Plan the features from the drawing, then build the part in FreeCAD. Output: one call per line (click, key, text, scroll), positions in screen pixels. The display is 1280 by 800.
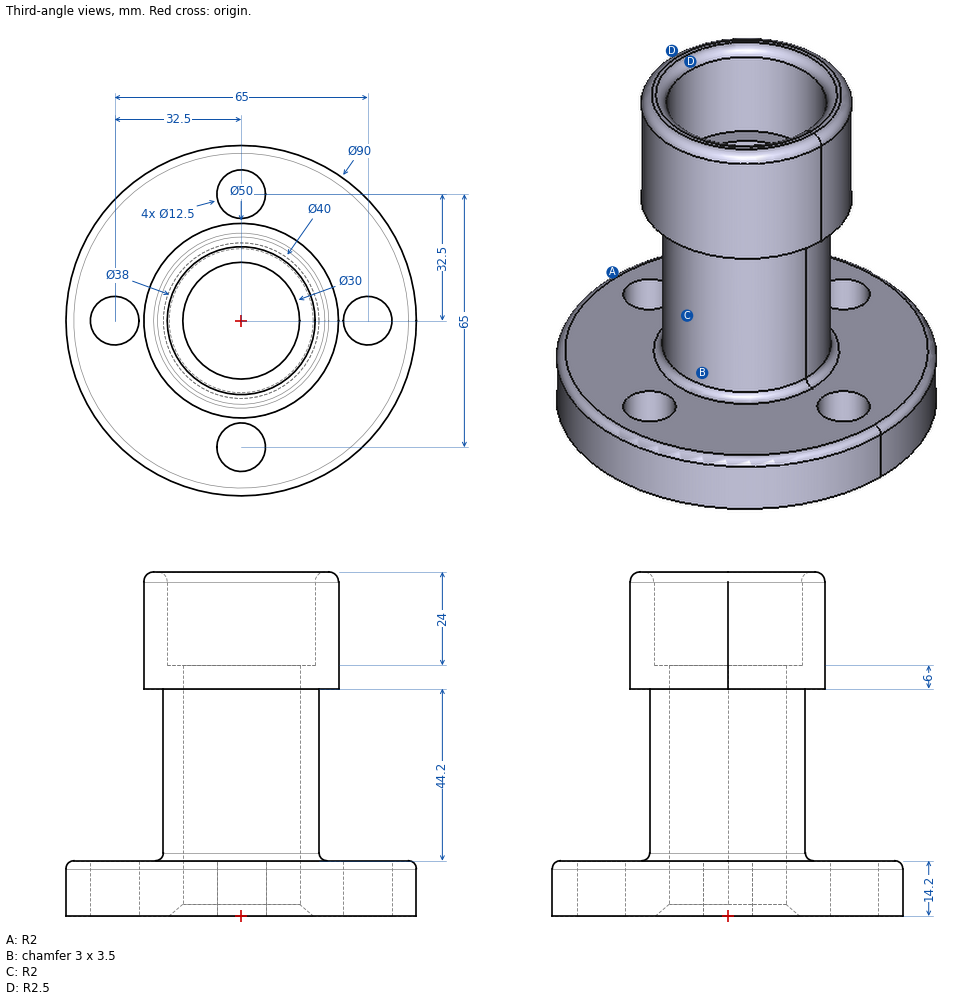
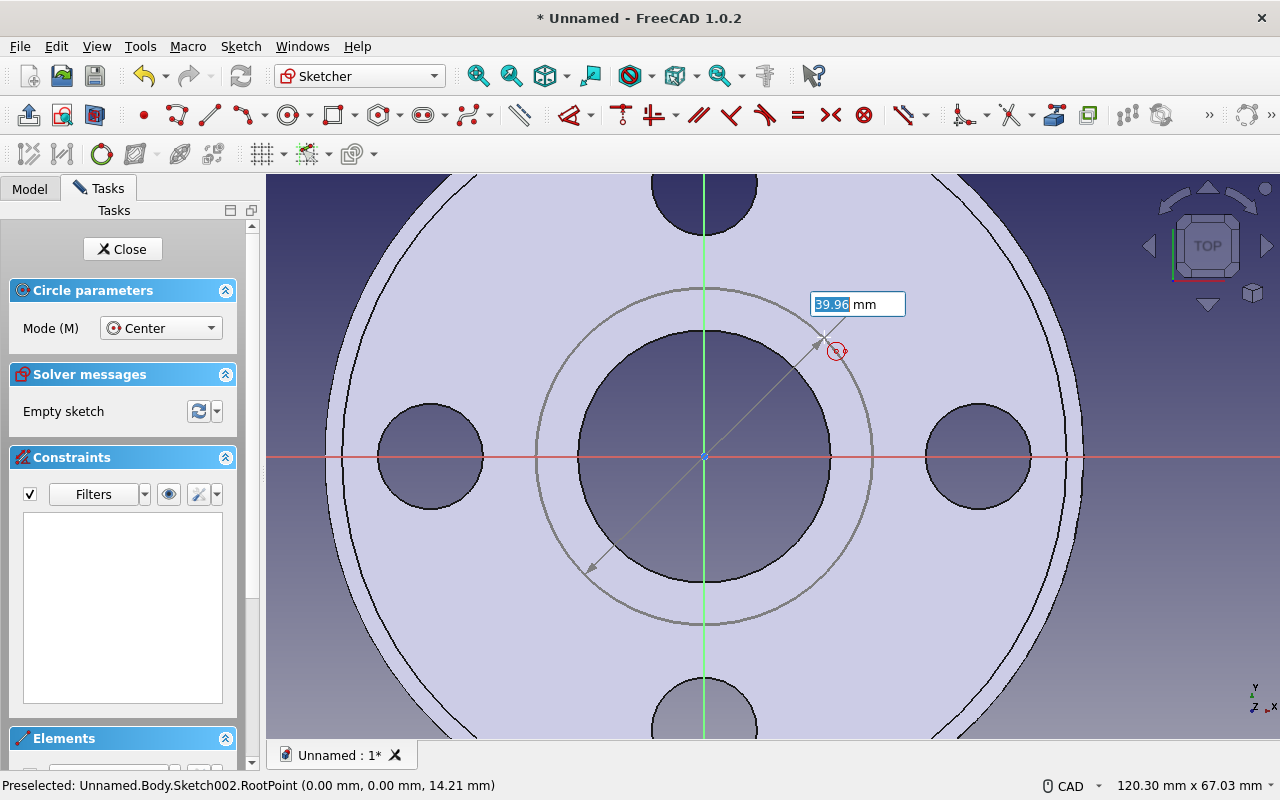
text(40)
key(Return)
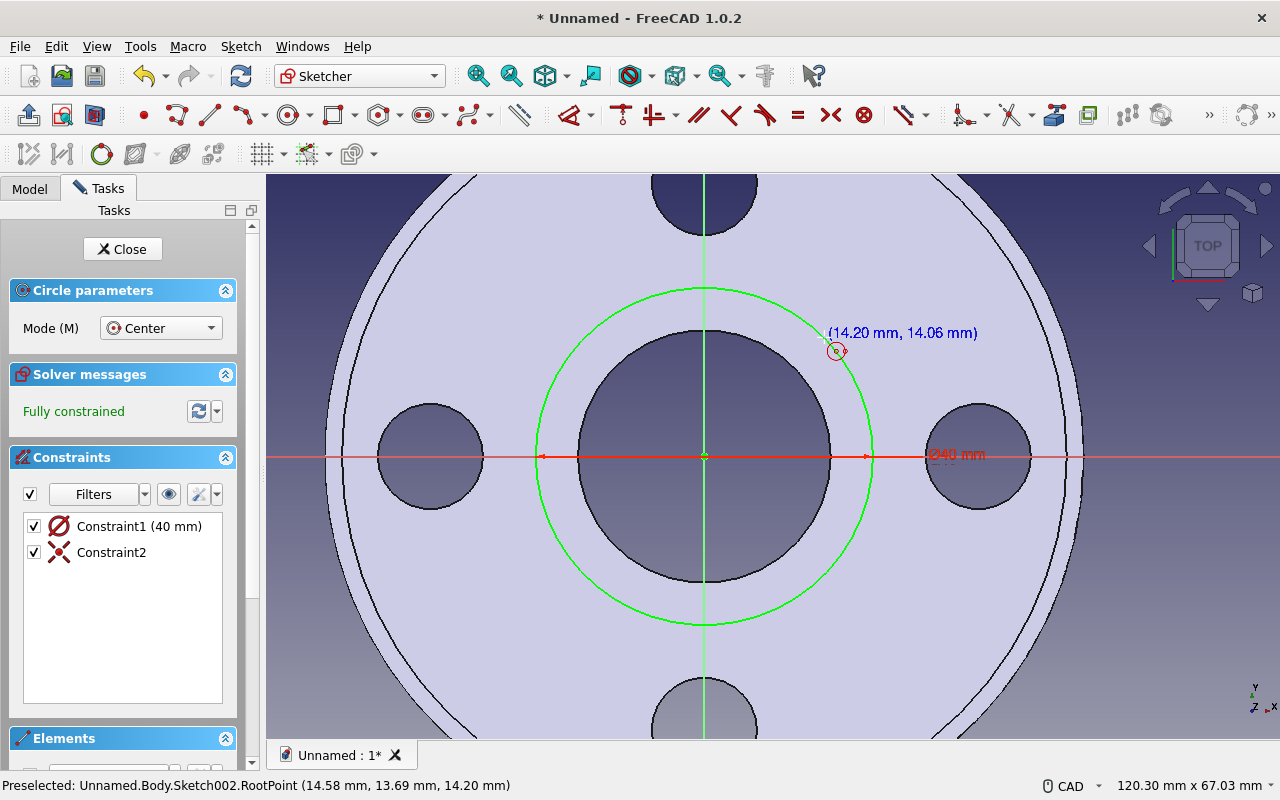
click(704, 456)
move(794, 367)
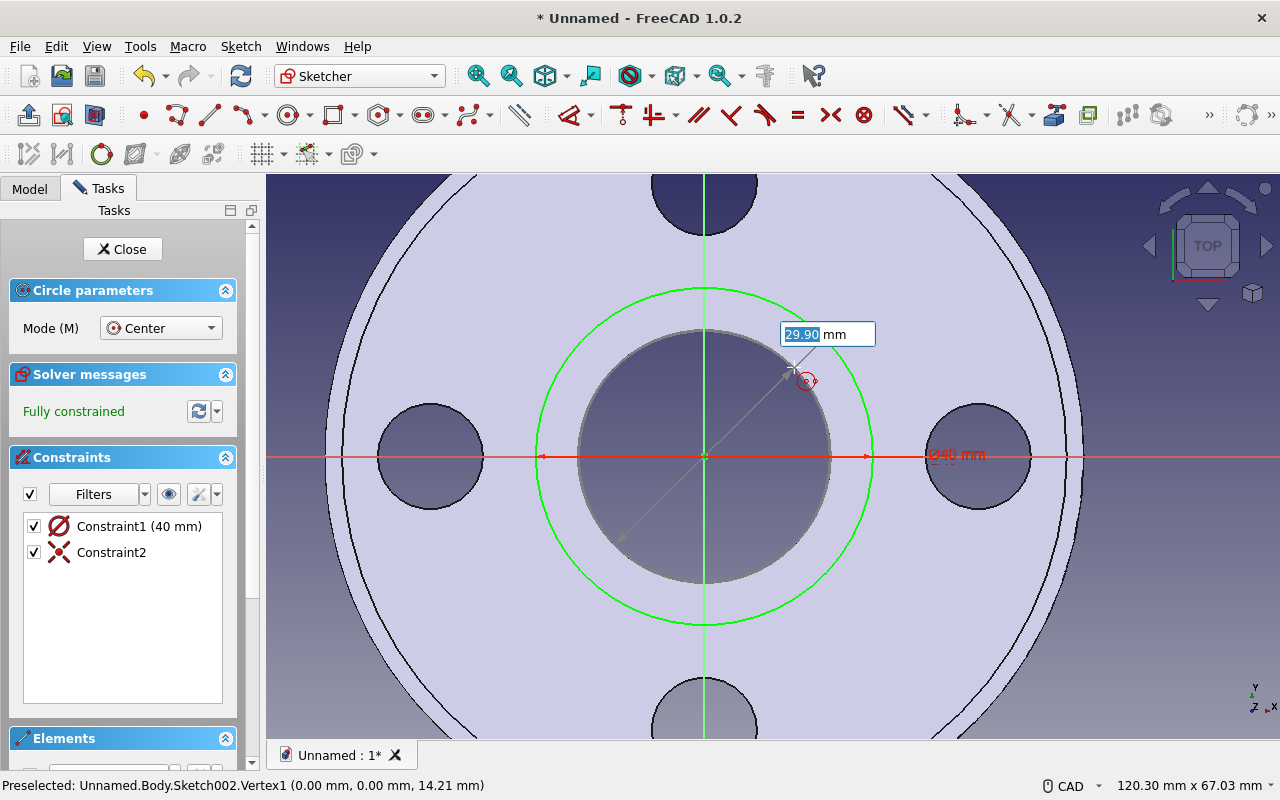
text(30)
key(Return)
key(Escape)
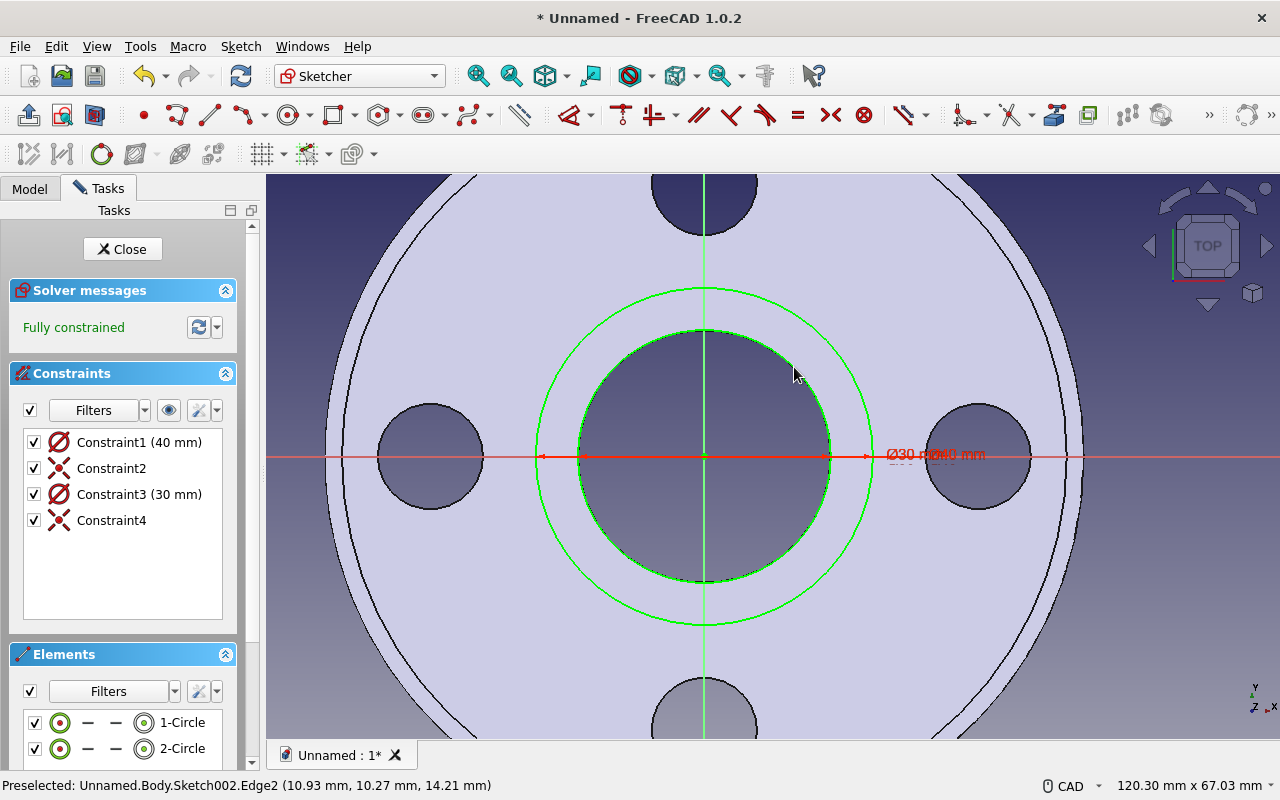
click(123, 249)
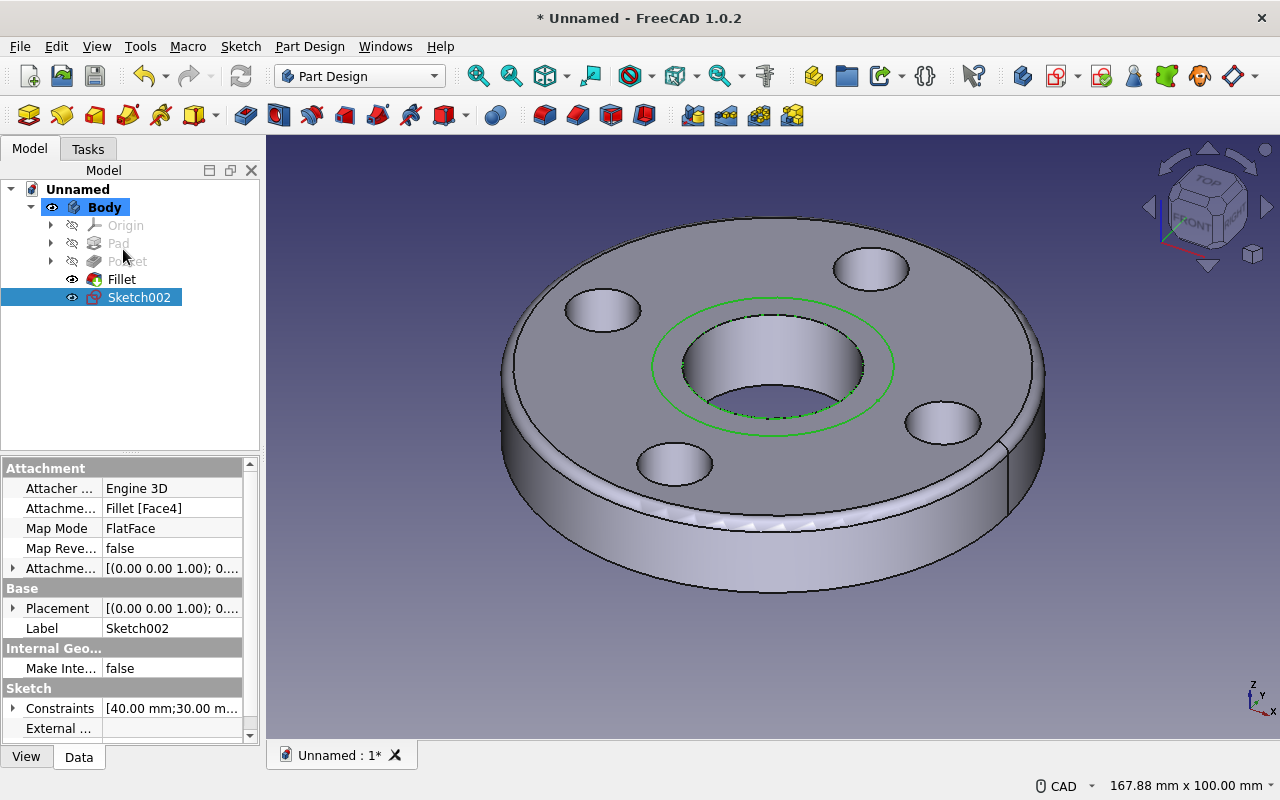
click(29, 116)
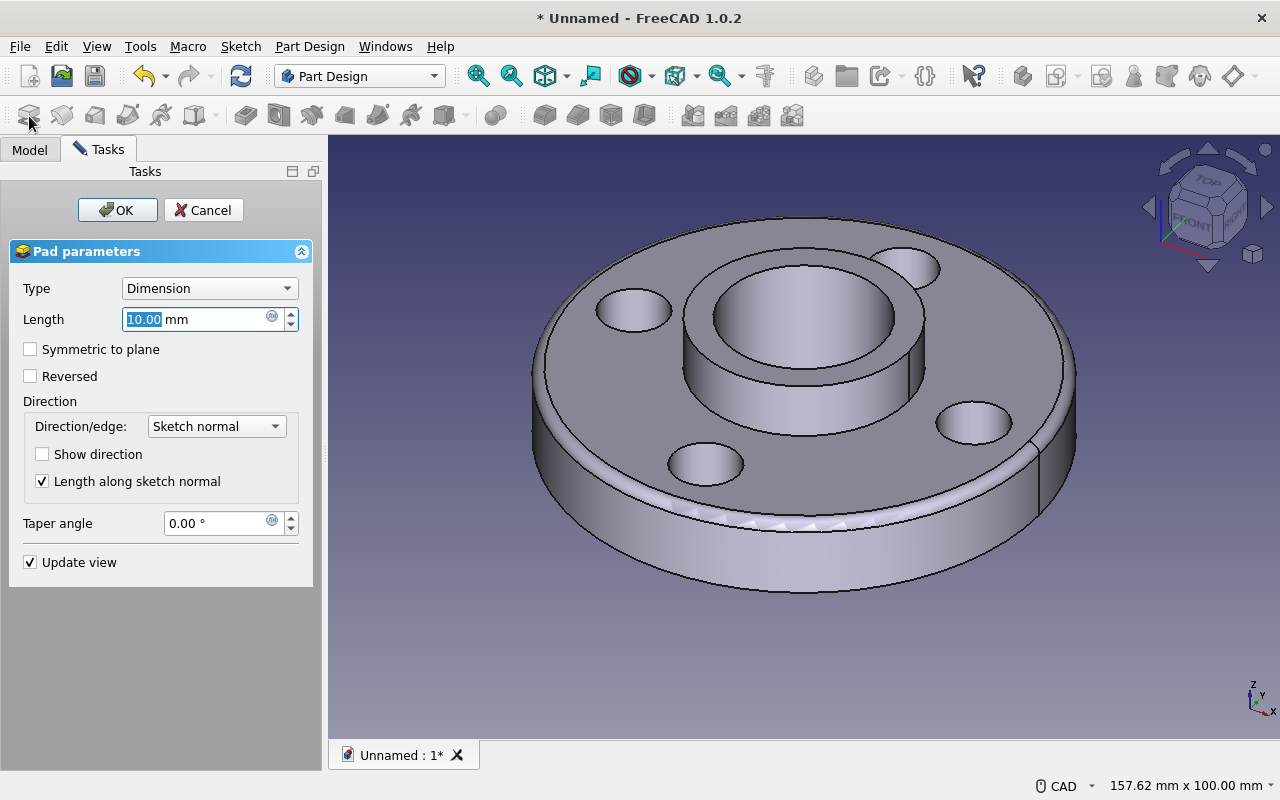
text(44.2)
key(Tab)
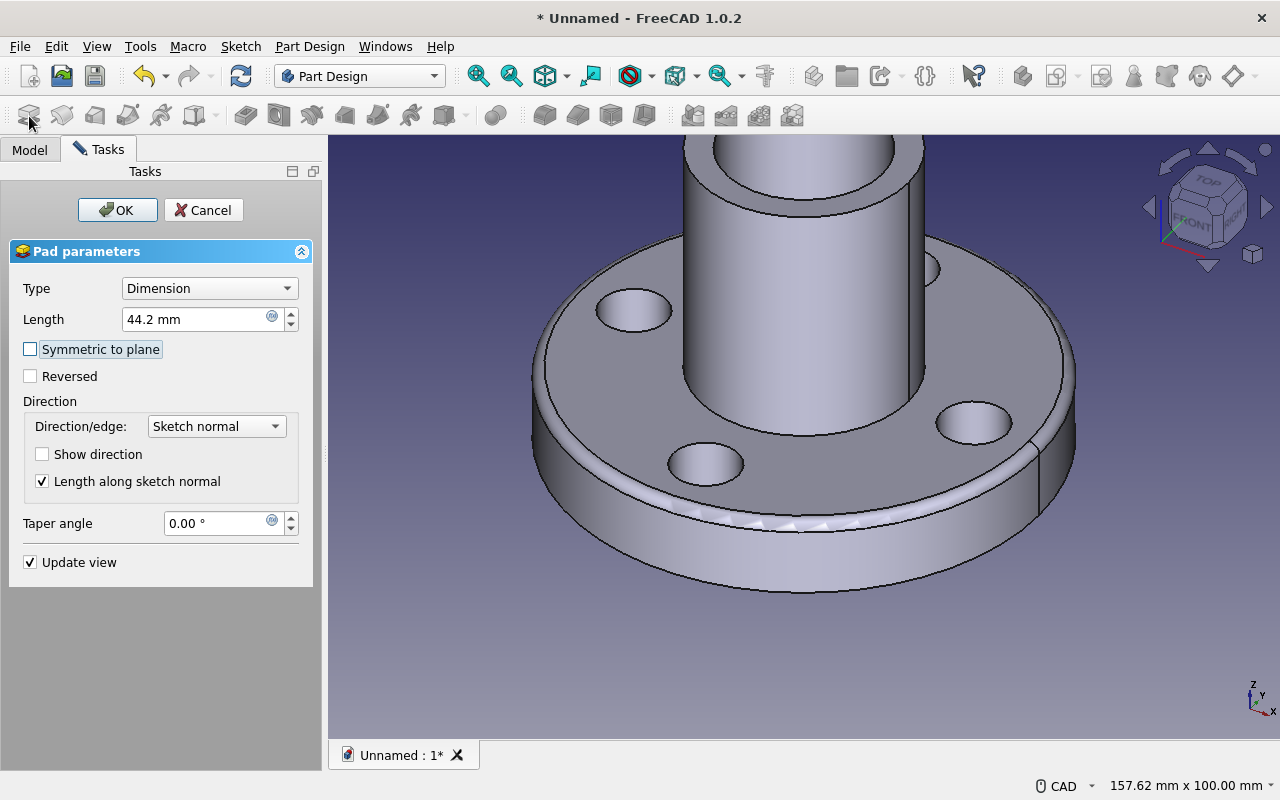
click(118, 210)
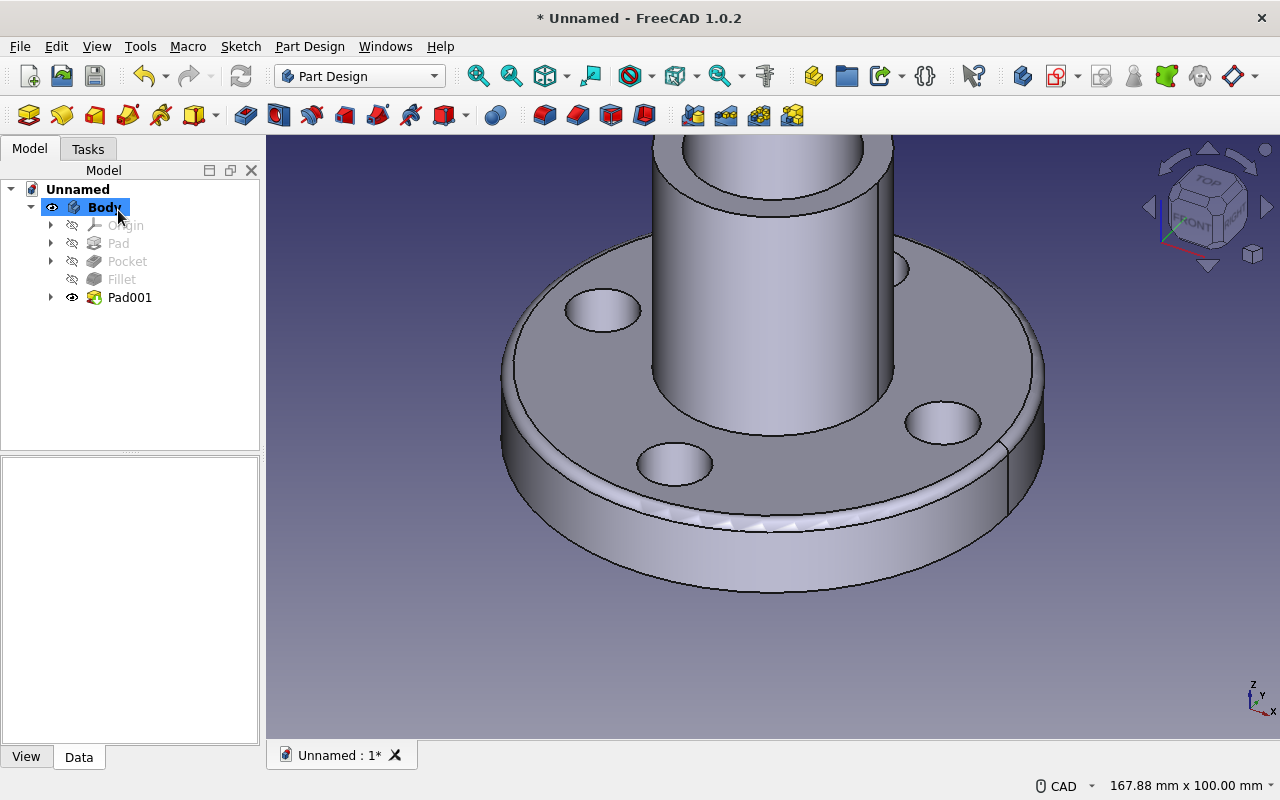
key(v)
key(f)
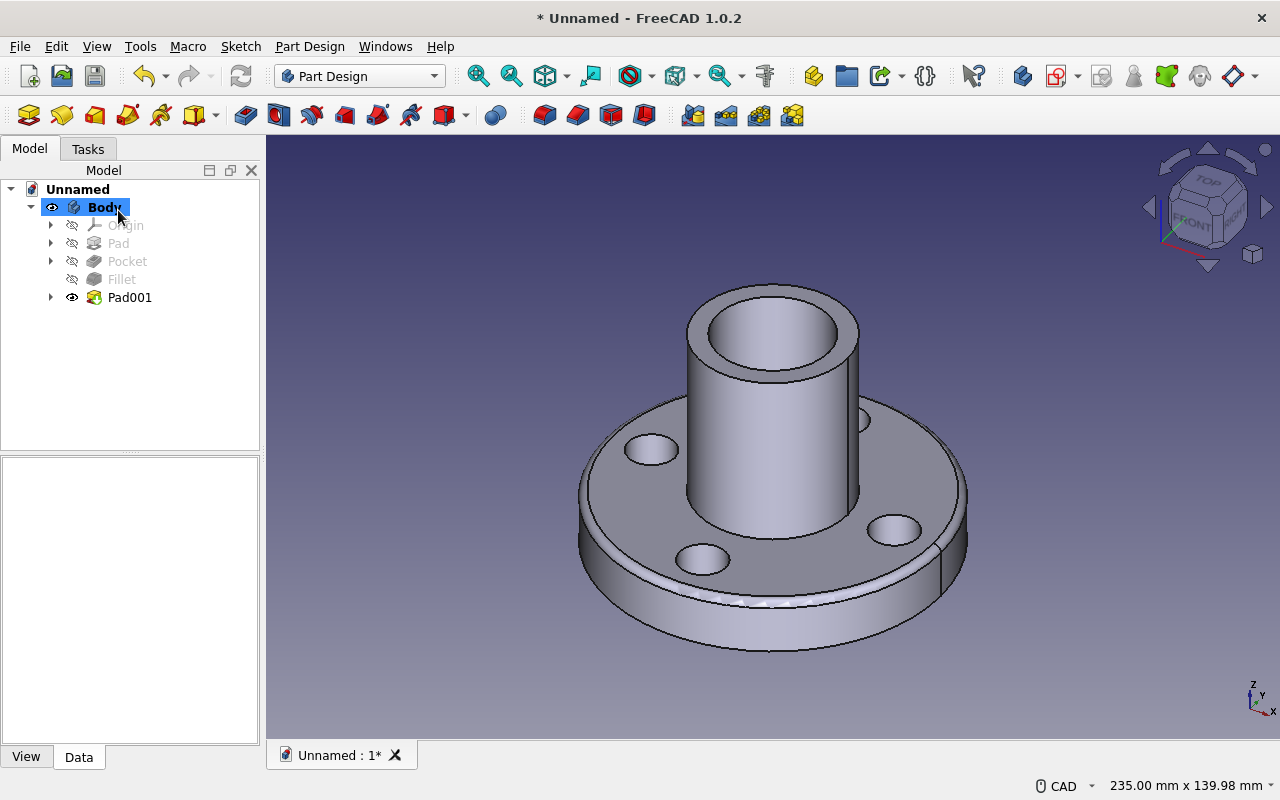
click(837, 354)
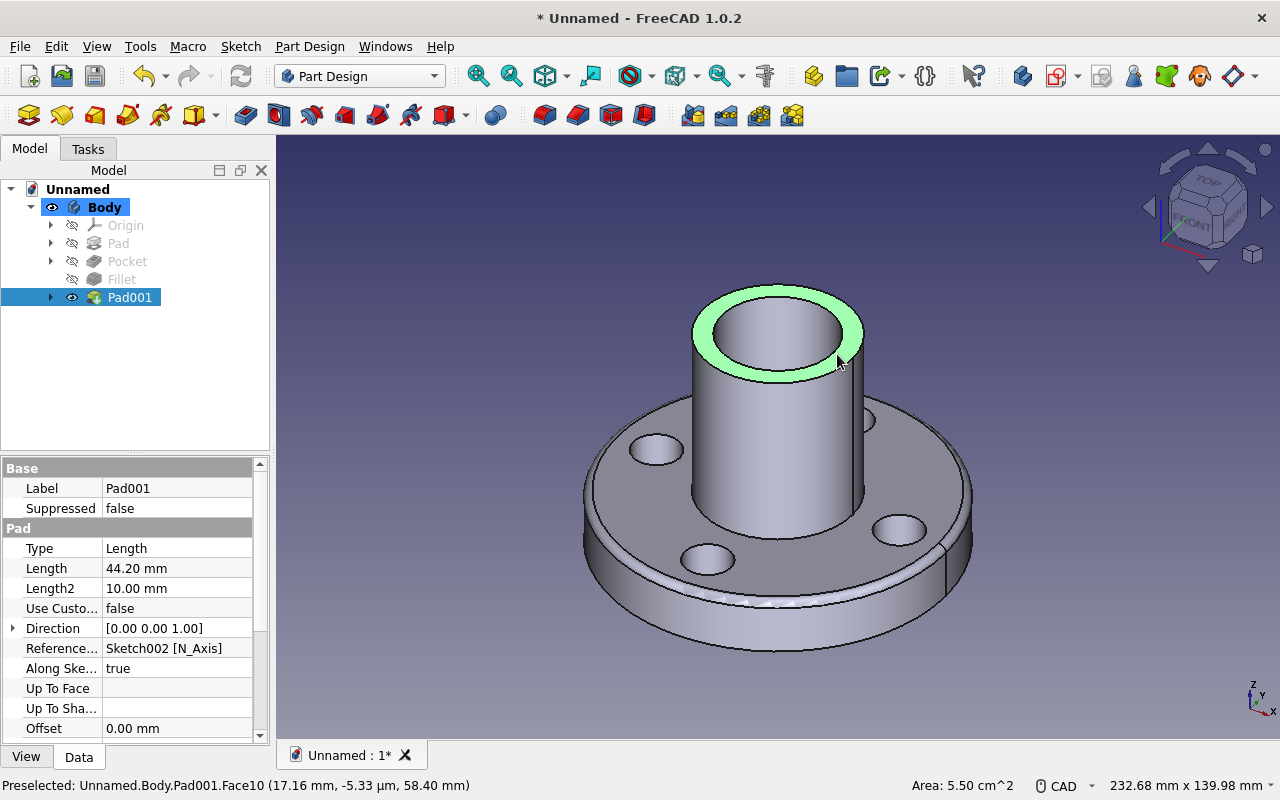
click(1056, 76)